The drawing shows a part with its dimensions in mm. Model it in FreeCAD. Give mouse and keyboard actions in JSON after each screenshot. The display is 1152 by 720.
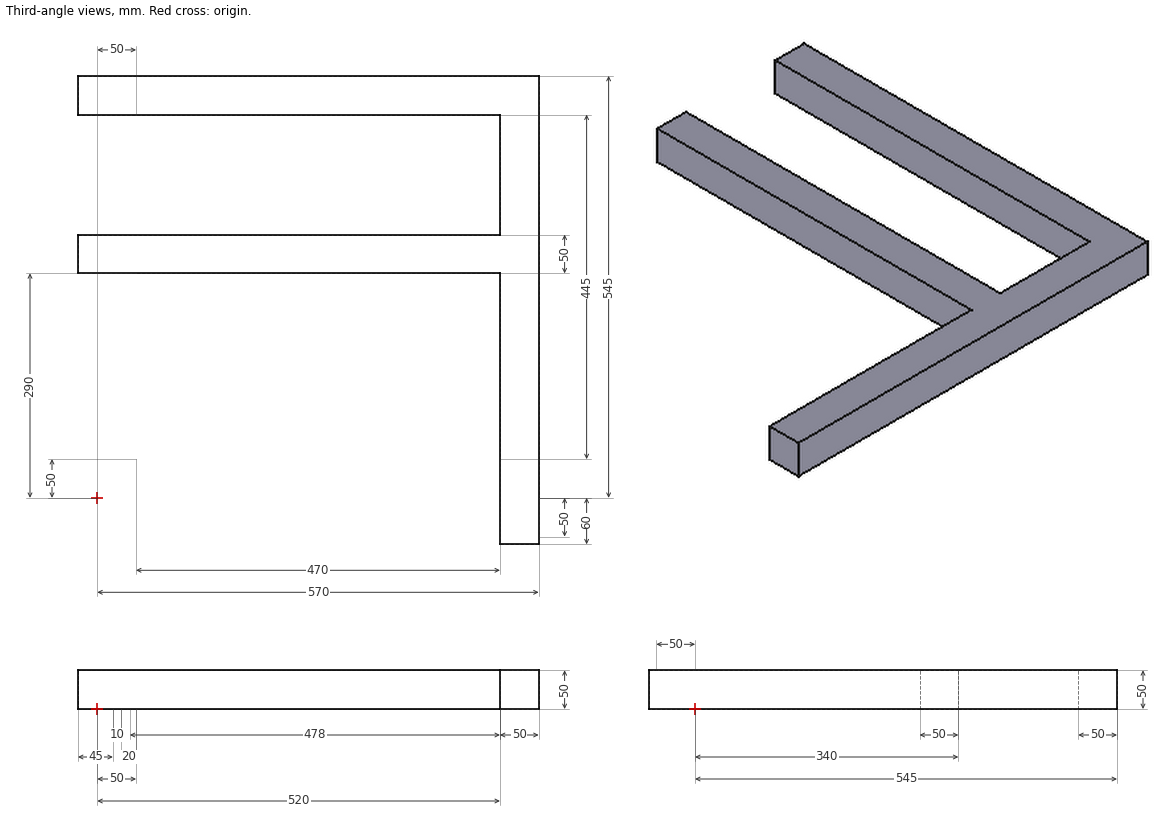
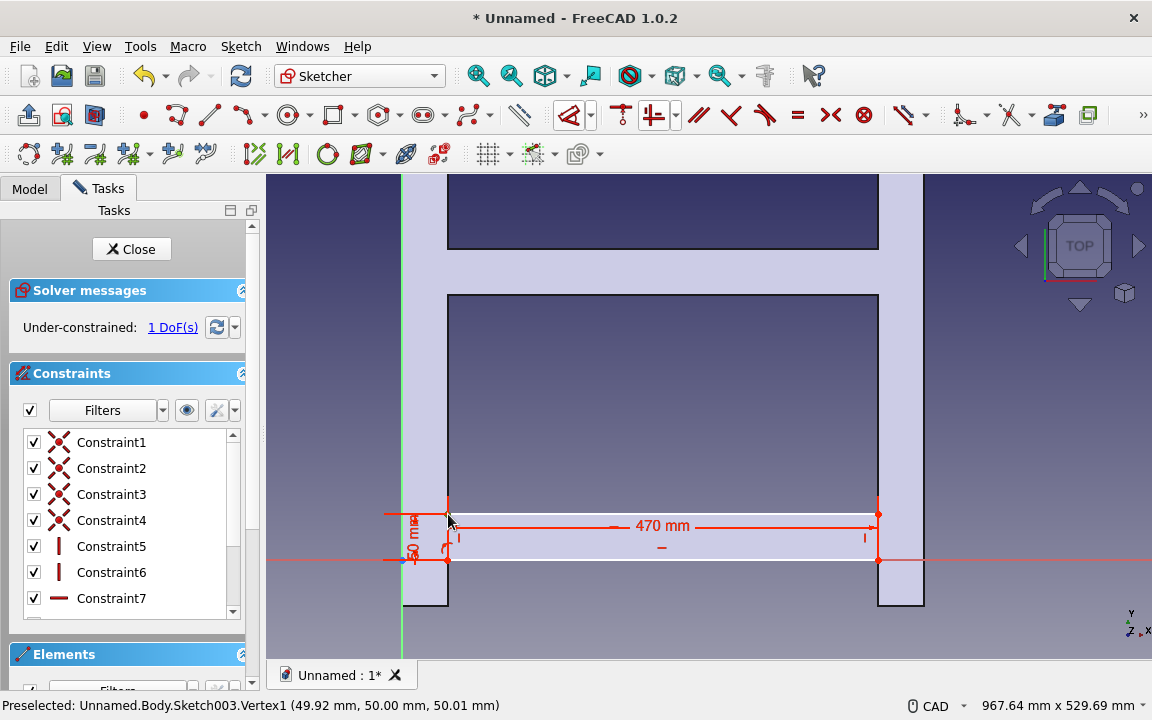
{"action": "key", "text": "l"}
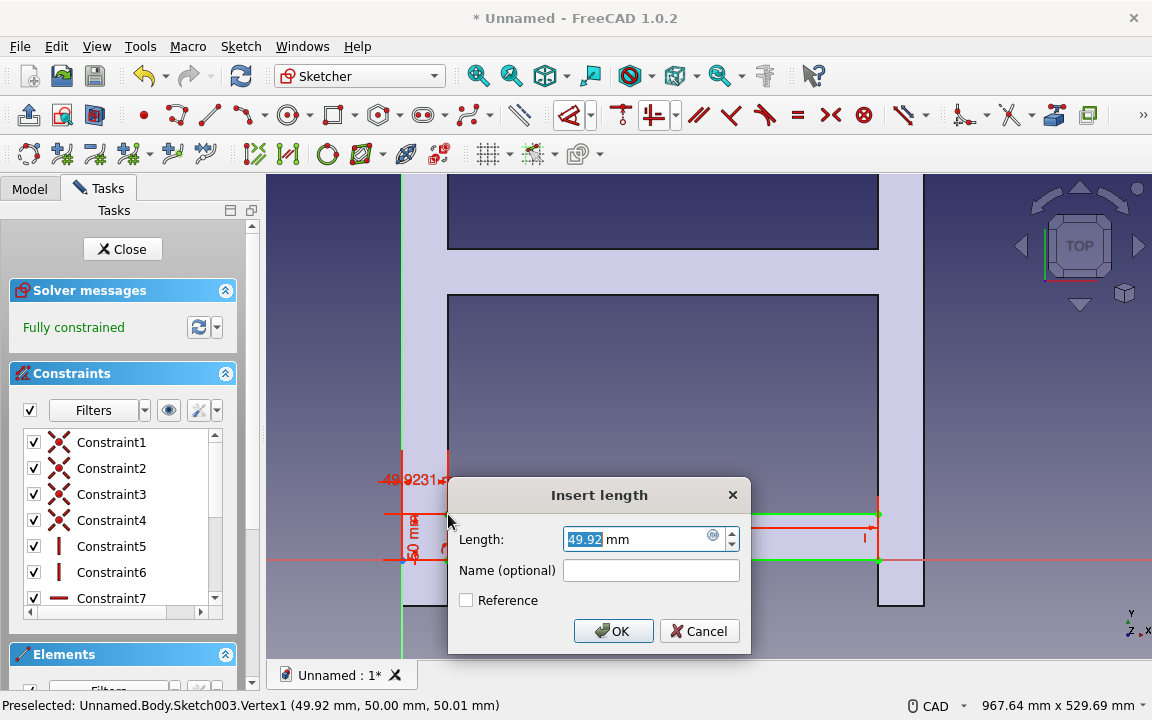
{"action": "type", "text": "50"}
{"action": "key", "text": "Return"}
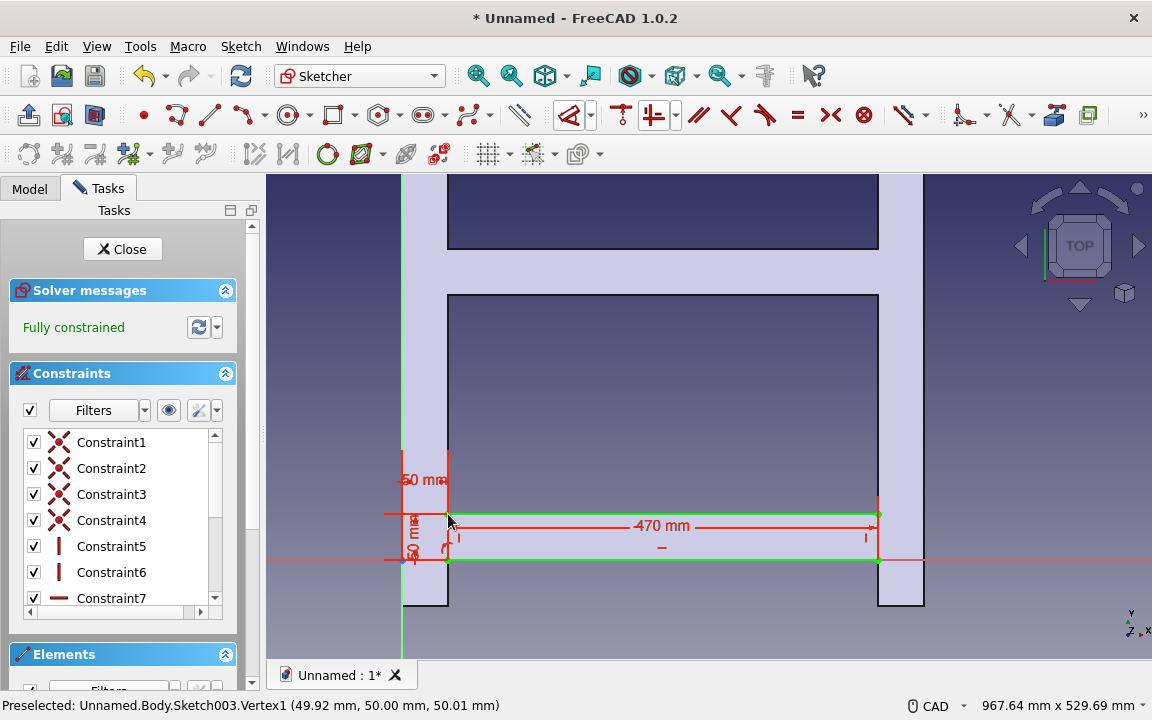
{"action": "left_click", "coordinate": [123, 249]}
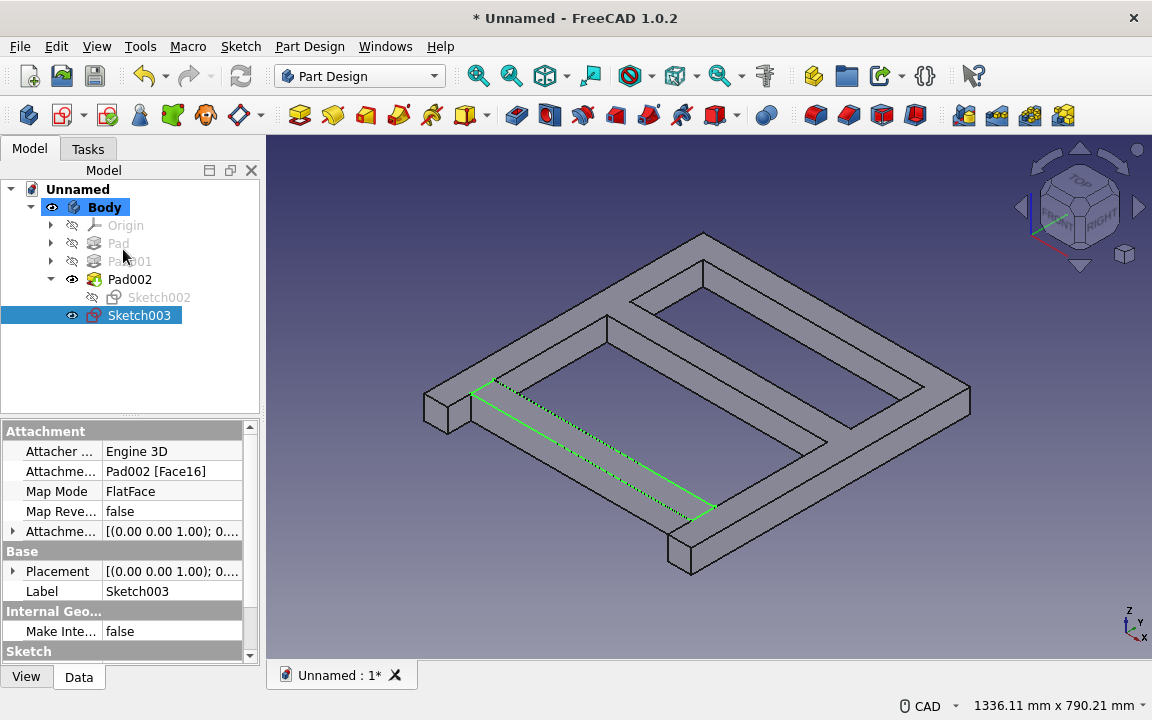
{"action": "left_click", "coordinate": [517, 116]}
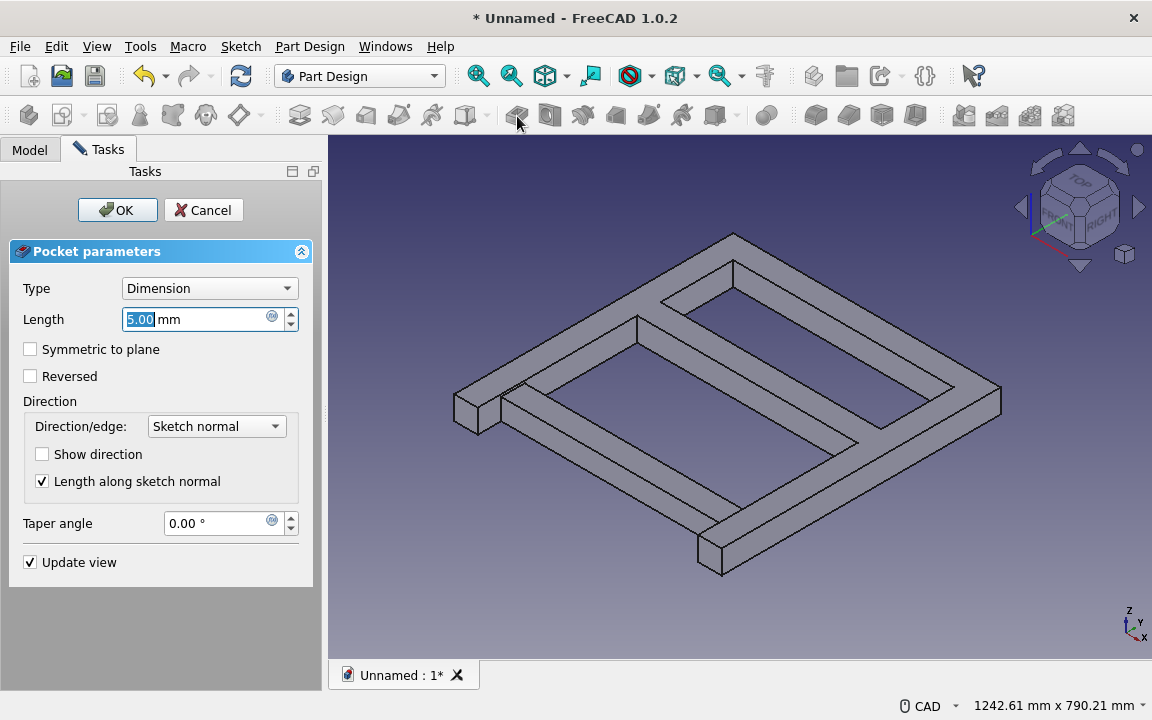
{"action": "type", "text": "50"}
{"action": "key", "text": "Tab"}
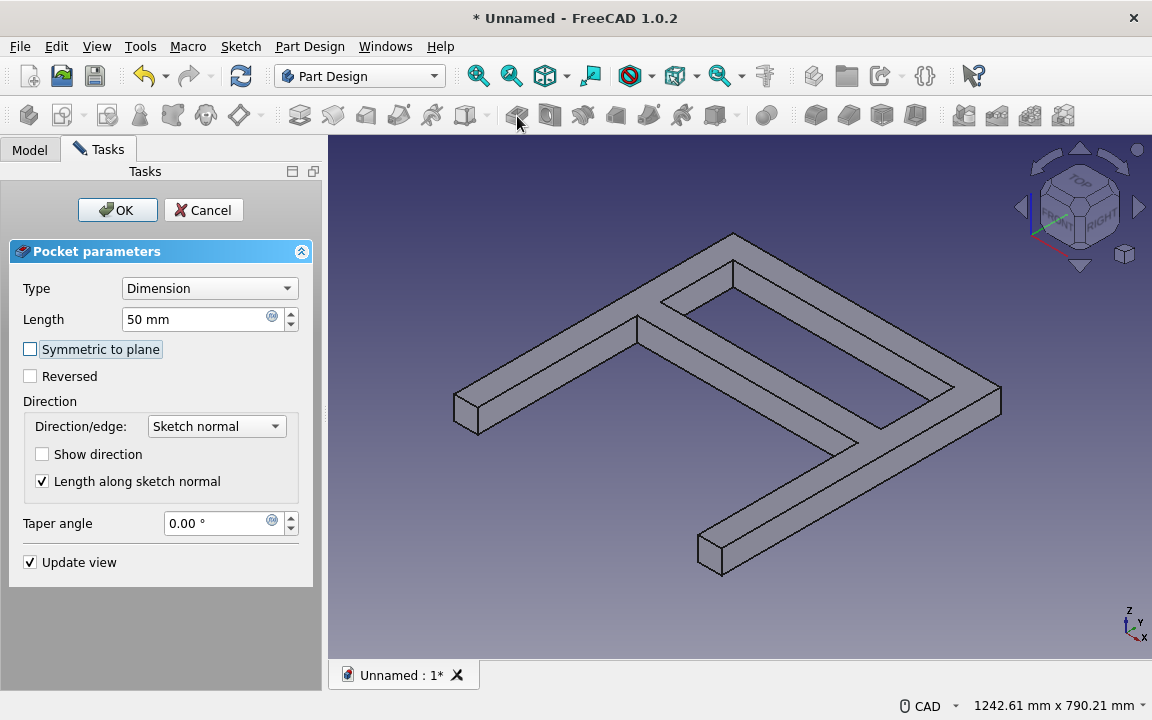
{"action": "left_click", "coordinate": [118, 210]}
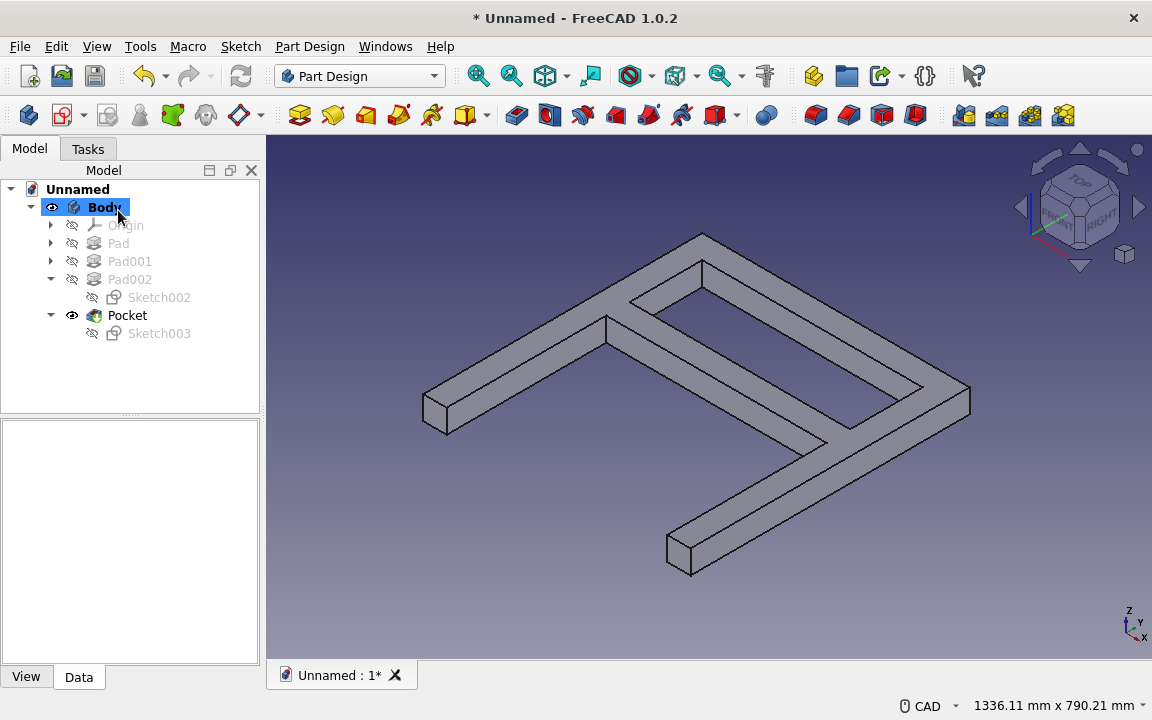
{"action": "left_click", "coordinate": [51, 225]}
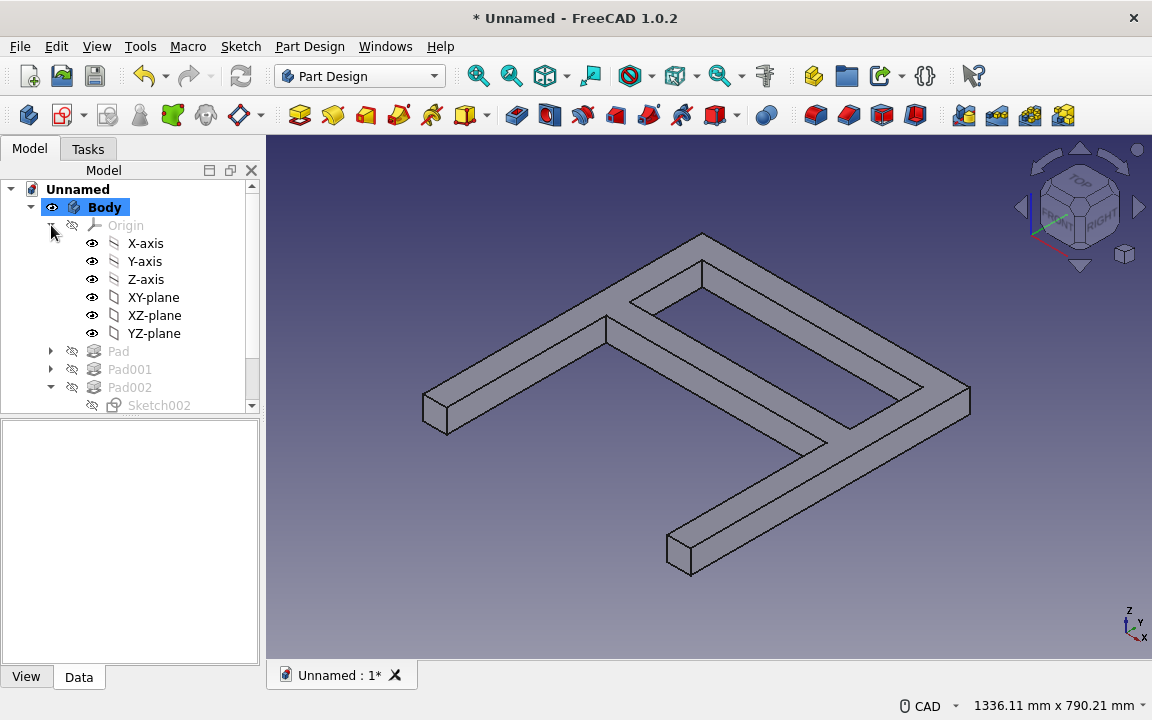
{"action": "left_click", "coordinate": [137, 333]}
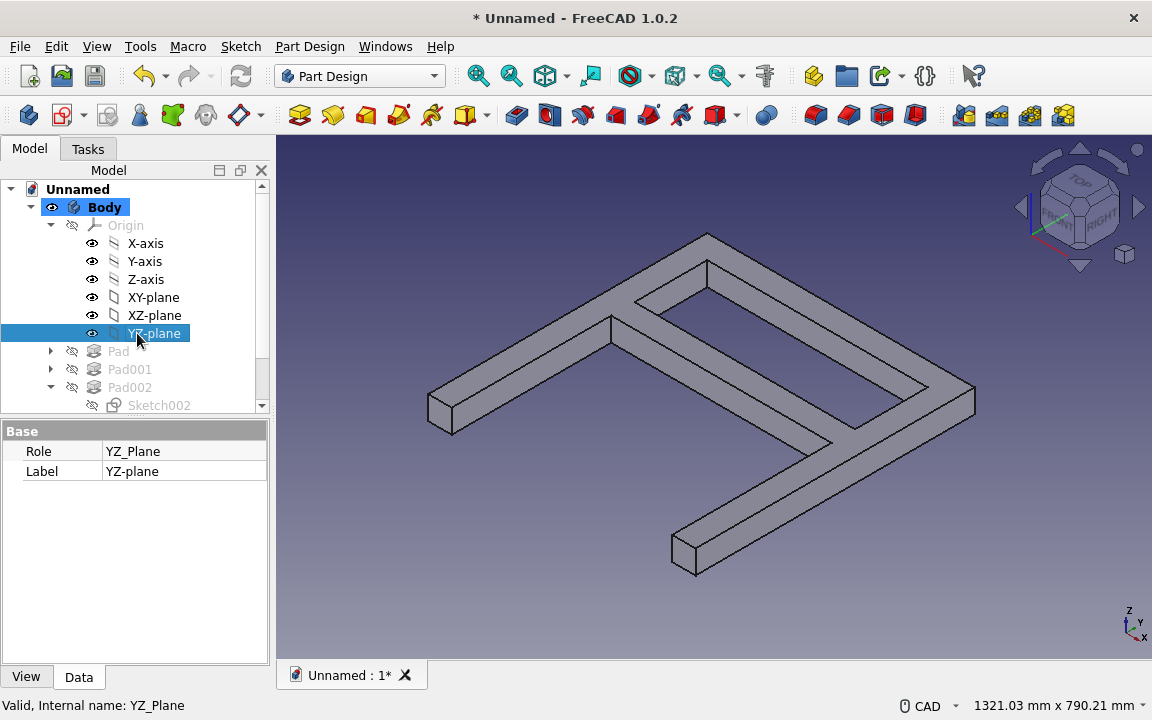
{"action": "left_click", "coordinate": [238, 116]}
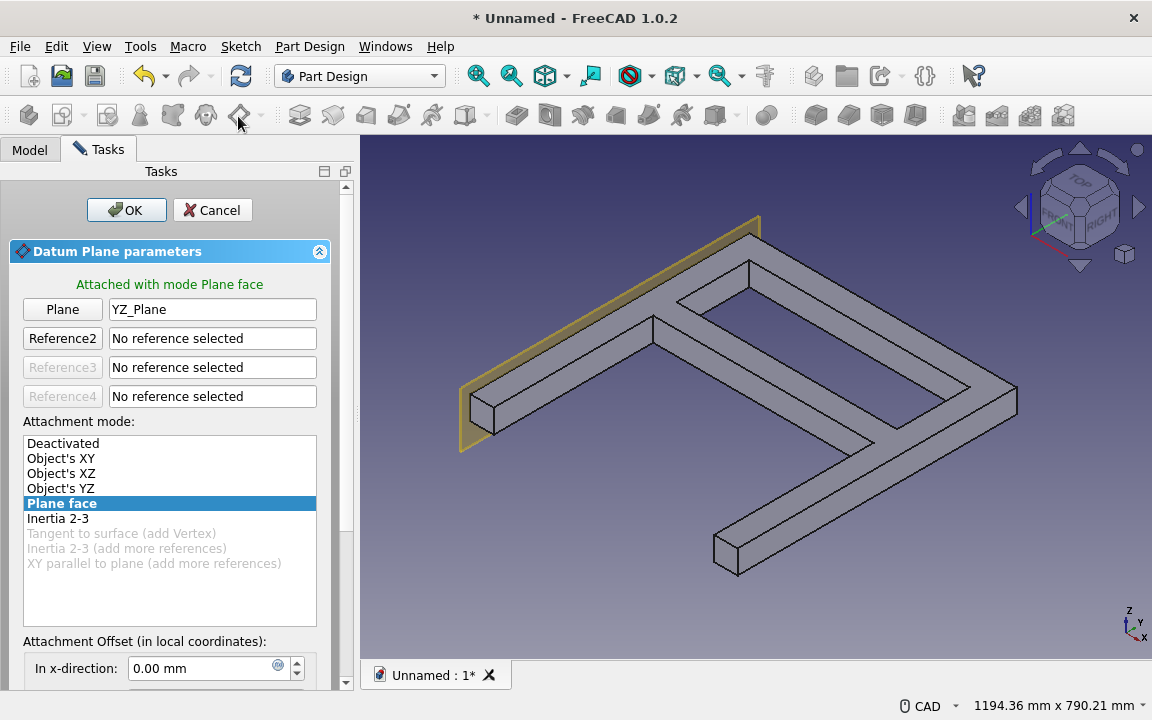
{"action": "scroll", "coordinate": [346, 436], "scroll_direction": "down", "scroll_amount": 2}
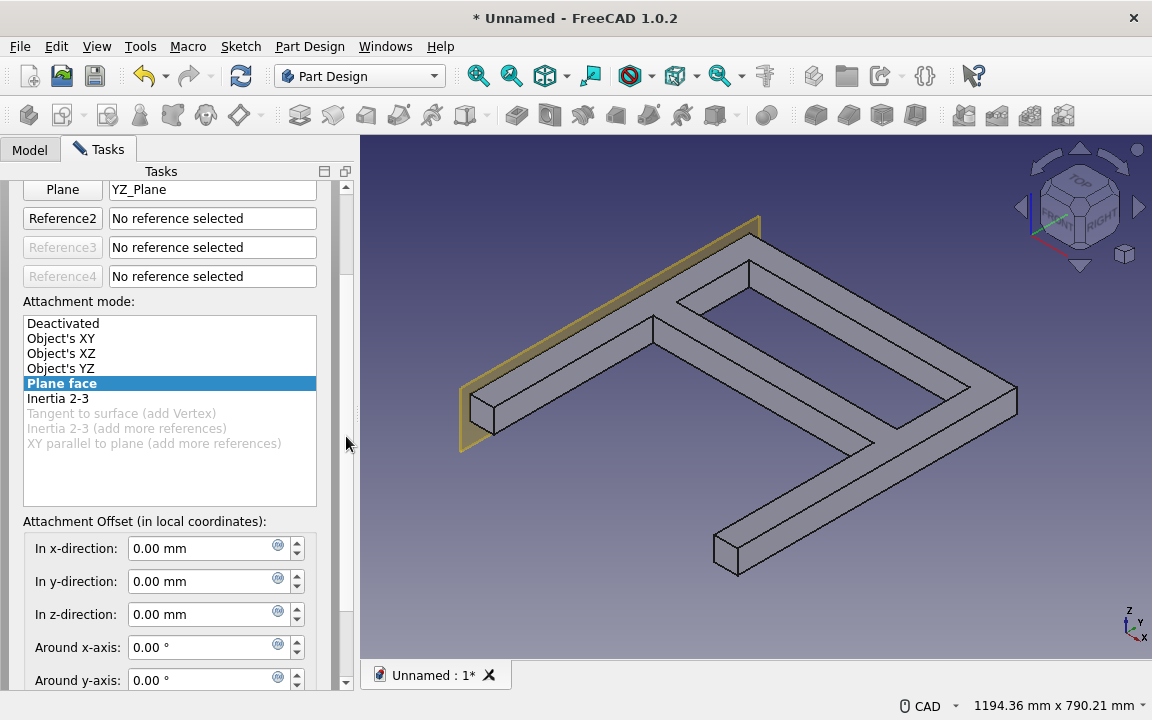
{"action": "triple_click", "coordinate": [210, 614]}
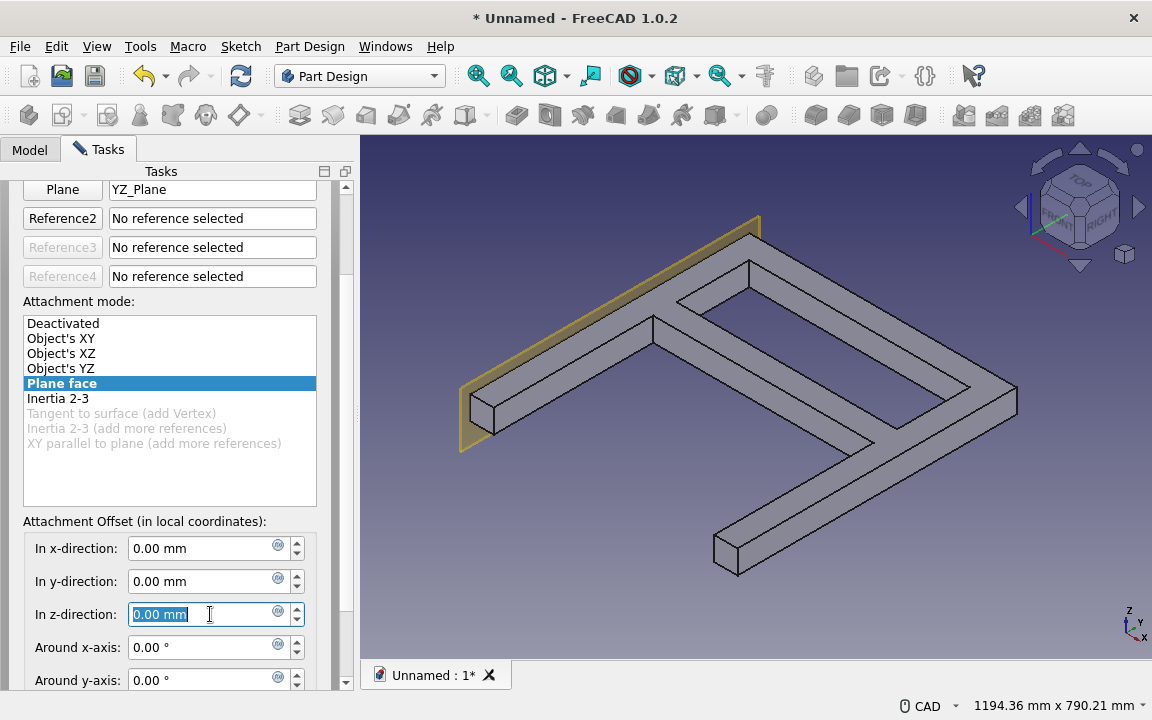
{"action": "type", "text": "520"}
{"action": "key", "text": "Tab"}